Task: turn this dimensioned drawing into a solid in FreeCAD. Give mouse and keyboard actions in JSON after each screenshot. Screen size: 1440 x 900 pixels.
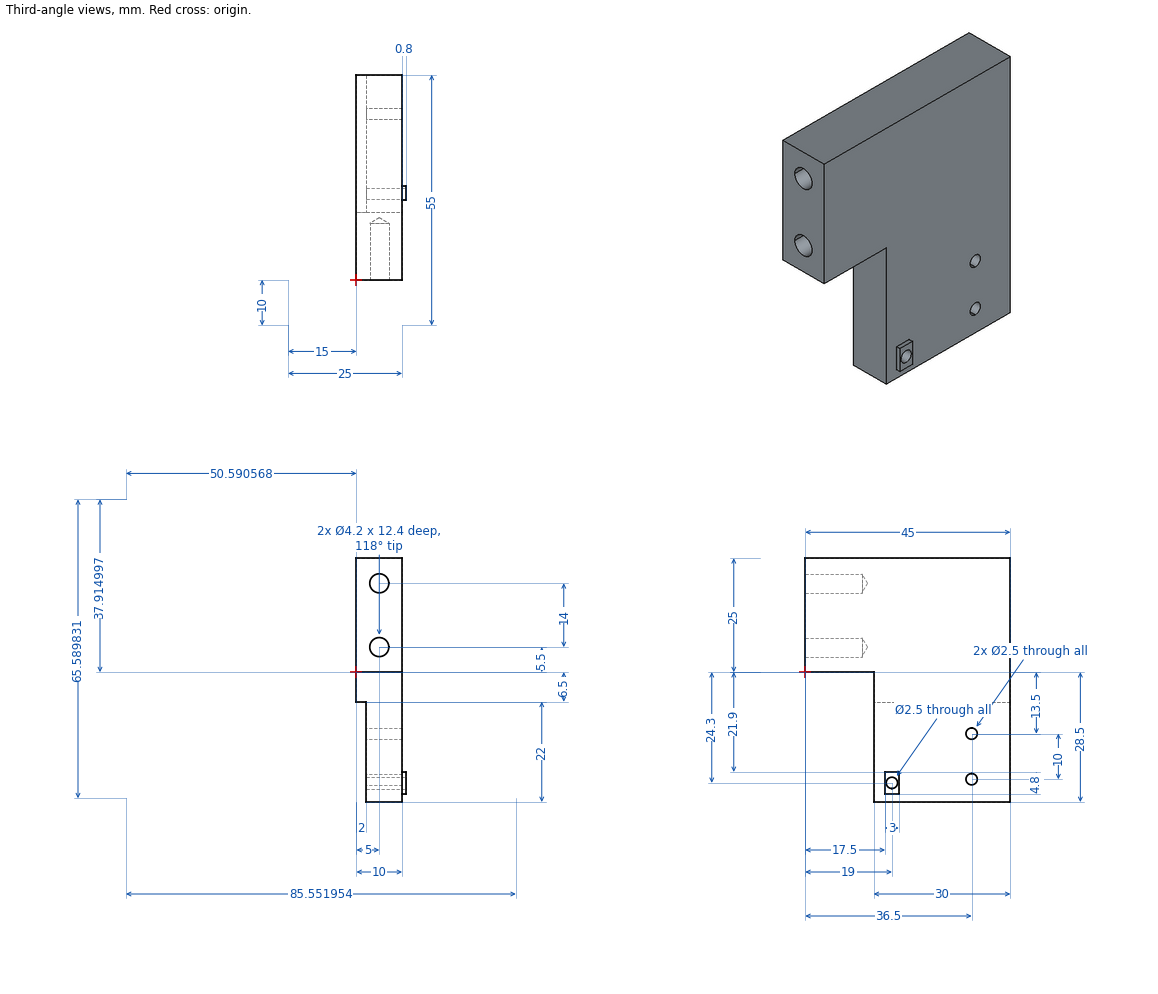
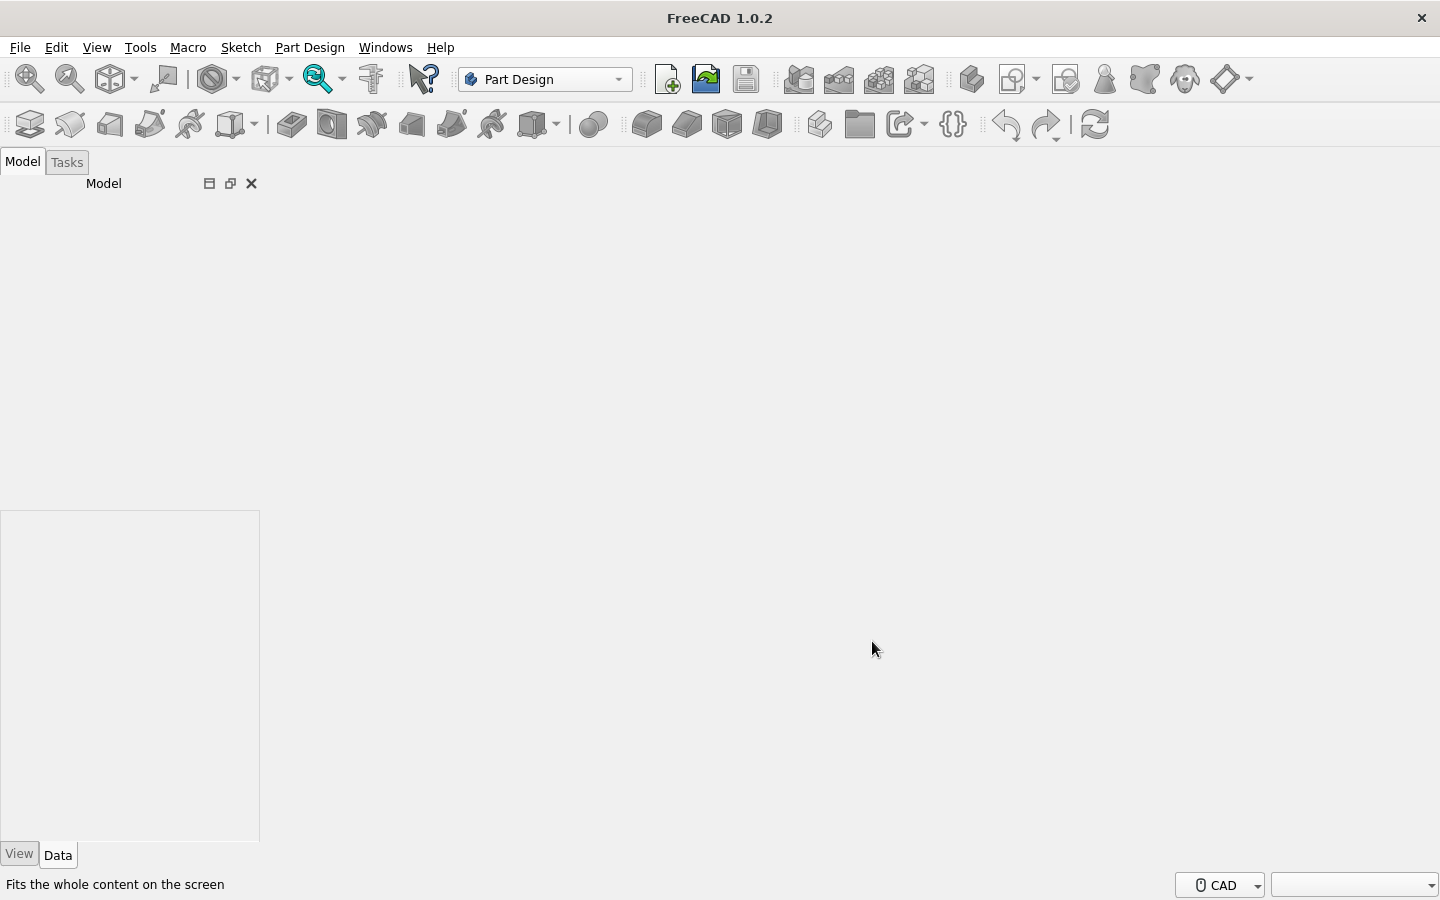
{"action": "left_click", "coordinate": [666, 80]}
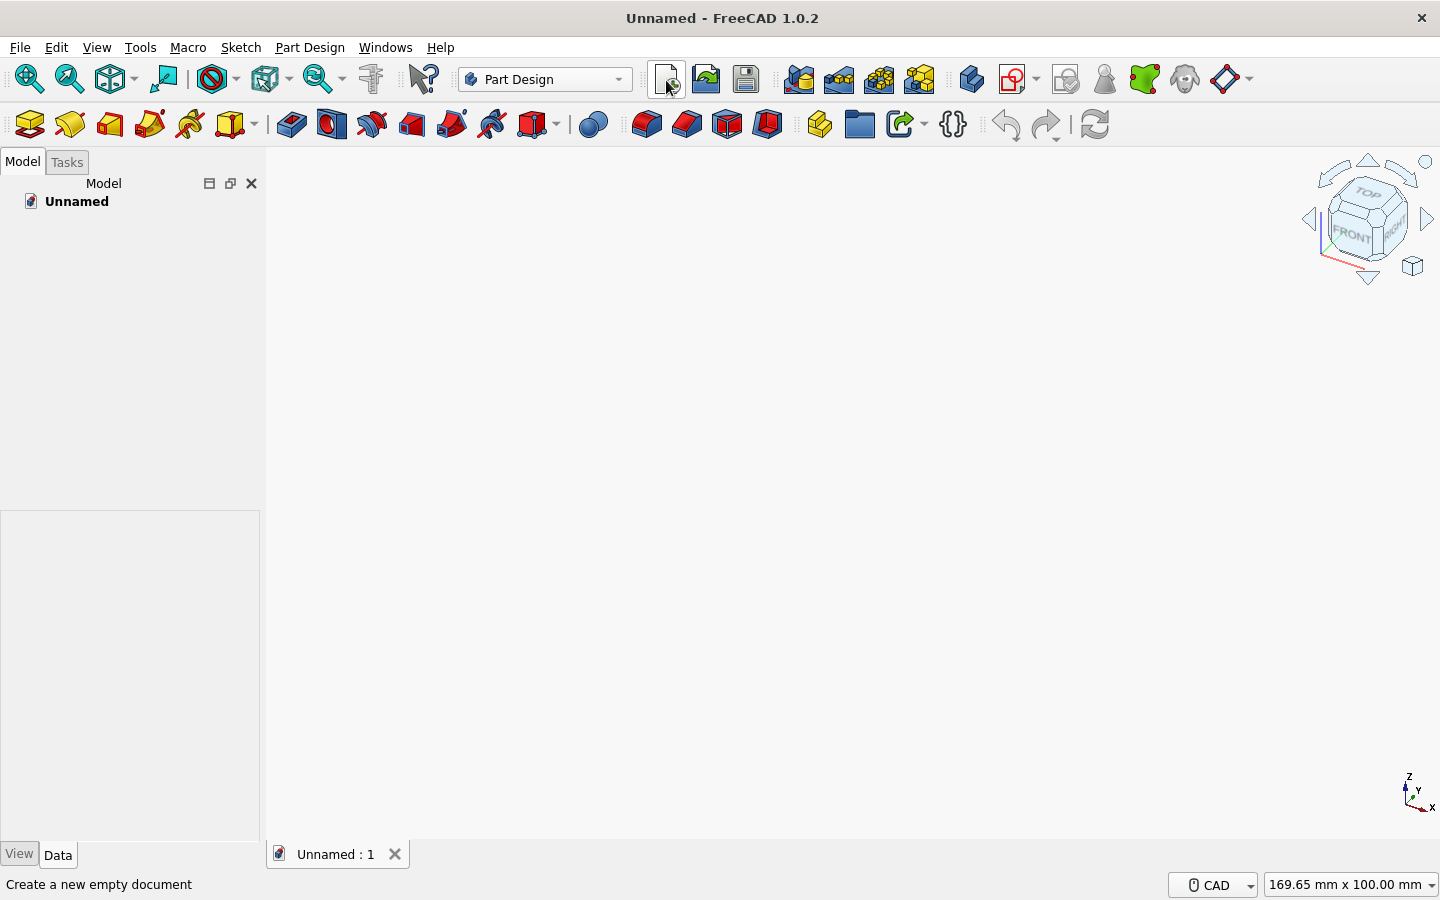
{"action": "left_click", "coordinate": [1012, 80]}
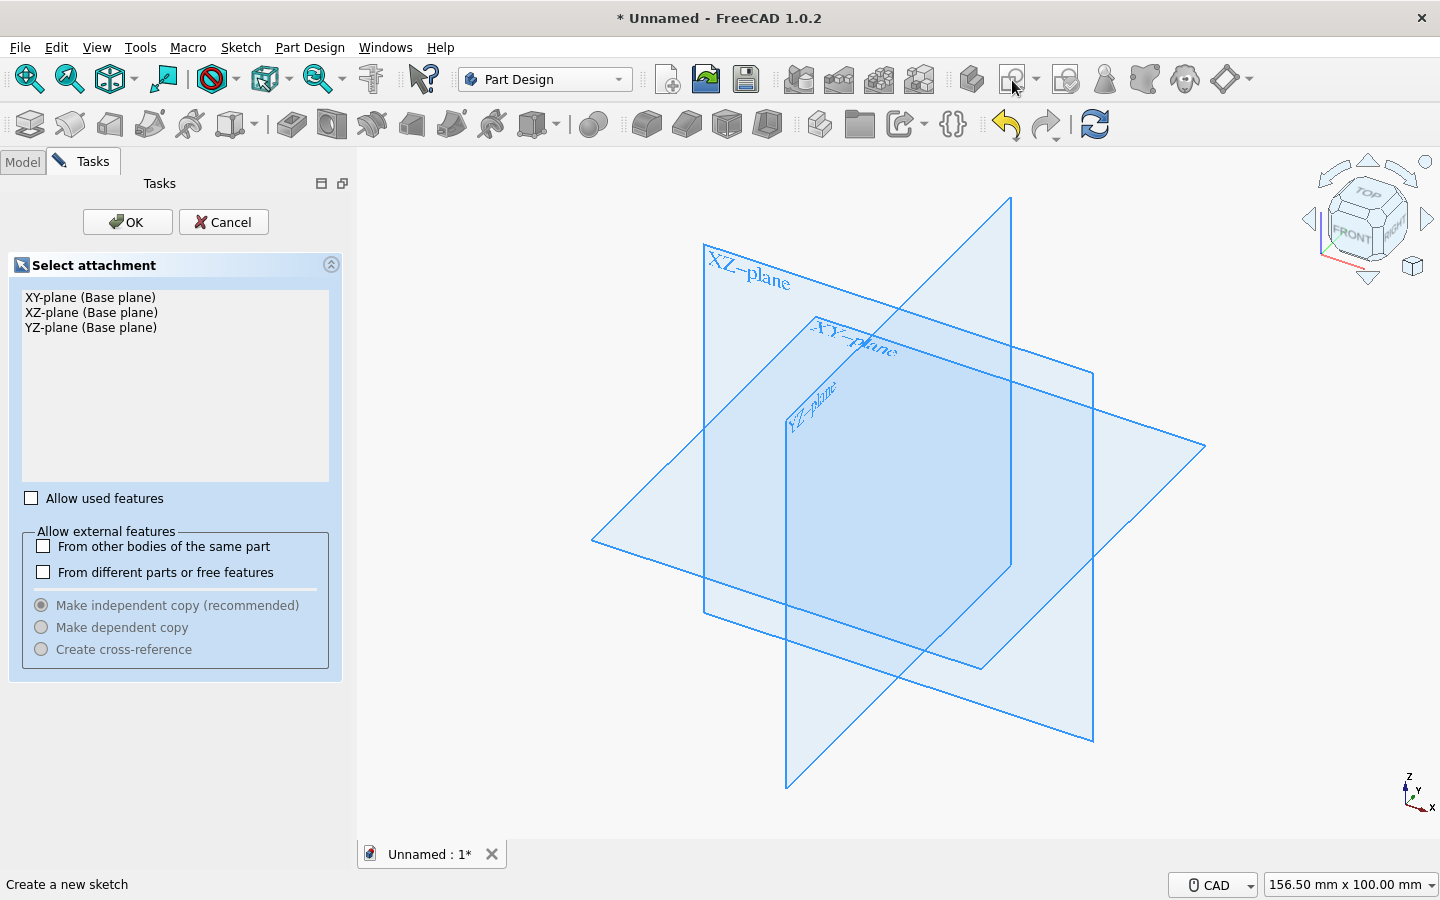
{"action": "left_click", "coordinate": [82, 298]}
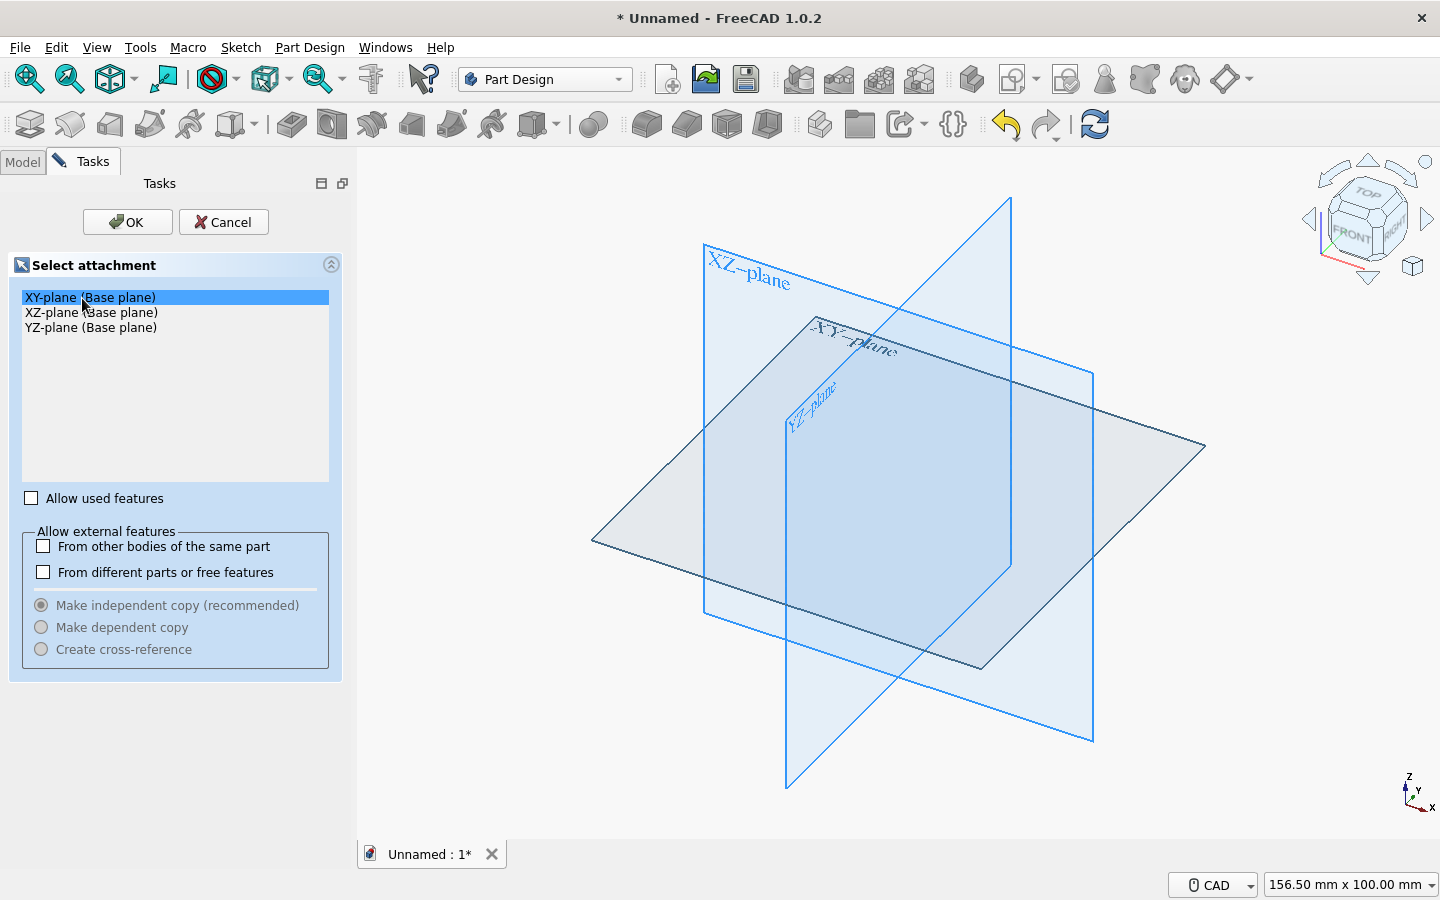
{"action": "left_click", "coordinate": [128, 222]}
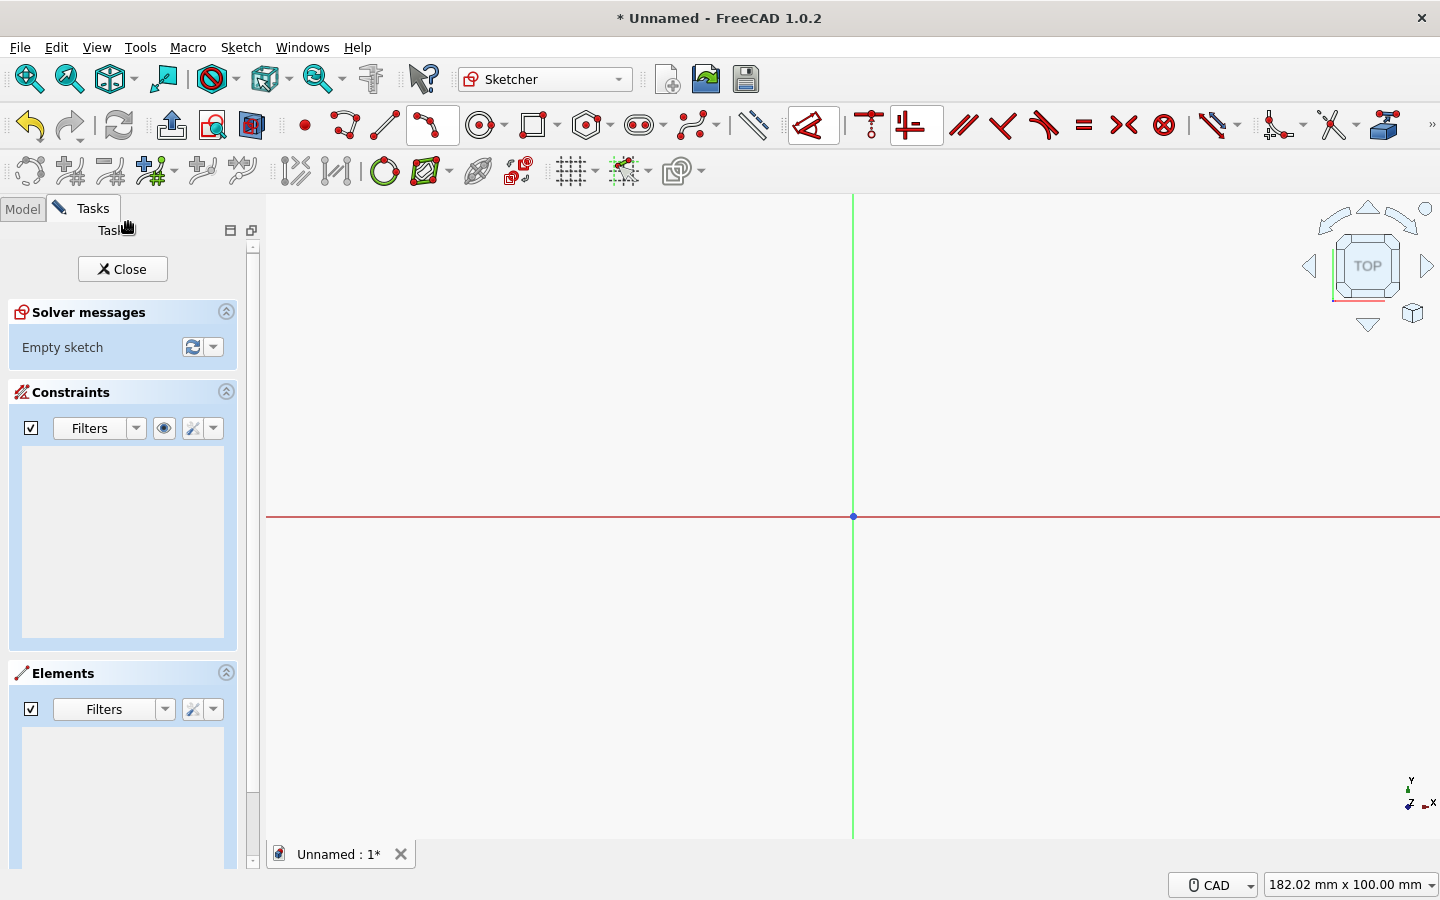
{"action": "scroll", "coordinate": [548, 811], "scroll_direction": "down", "scroll_amount": 1}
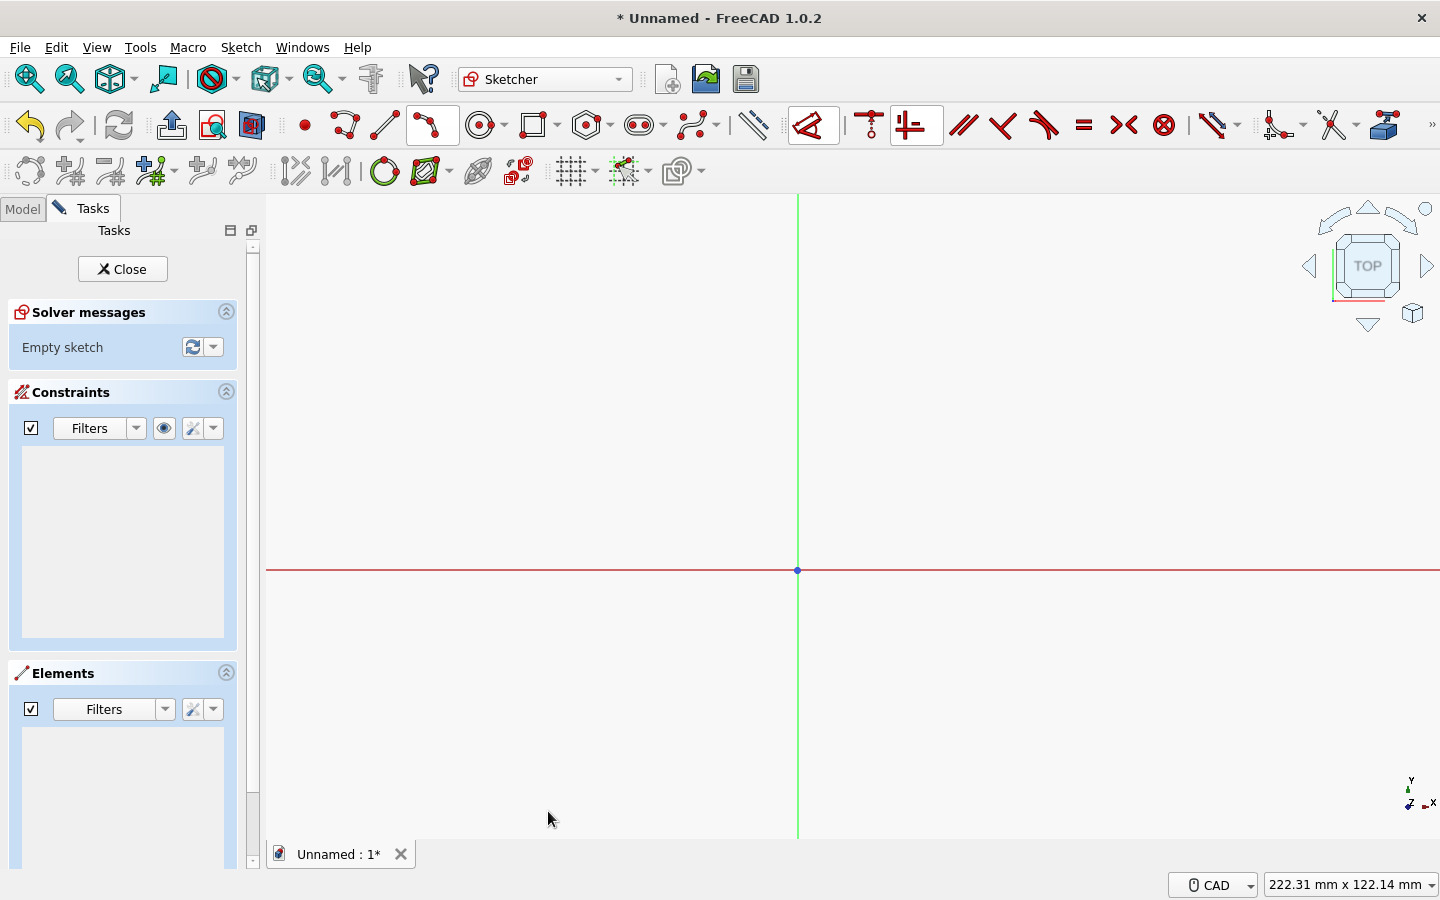
{"action": "scroll", "coordinate": [785, 399], "scroll_direction": "up", "scroll_amount": 2}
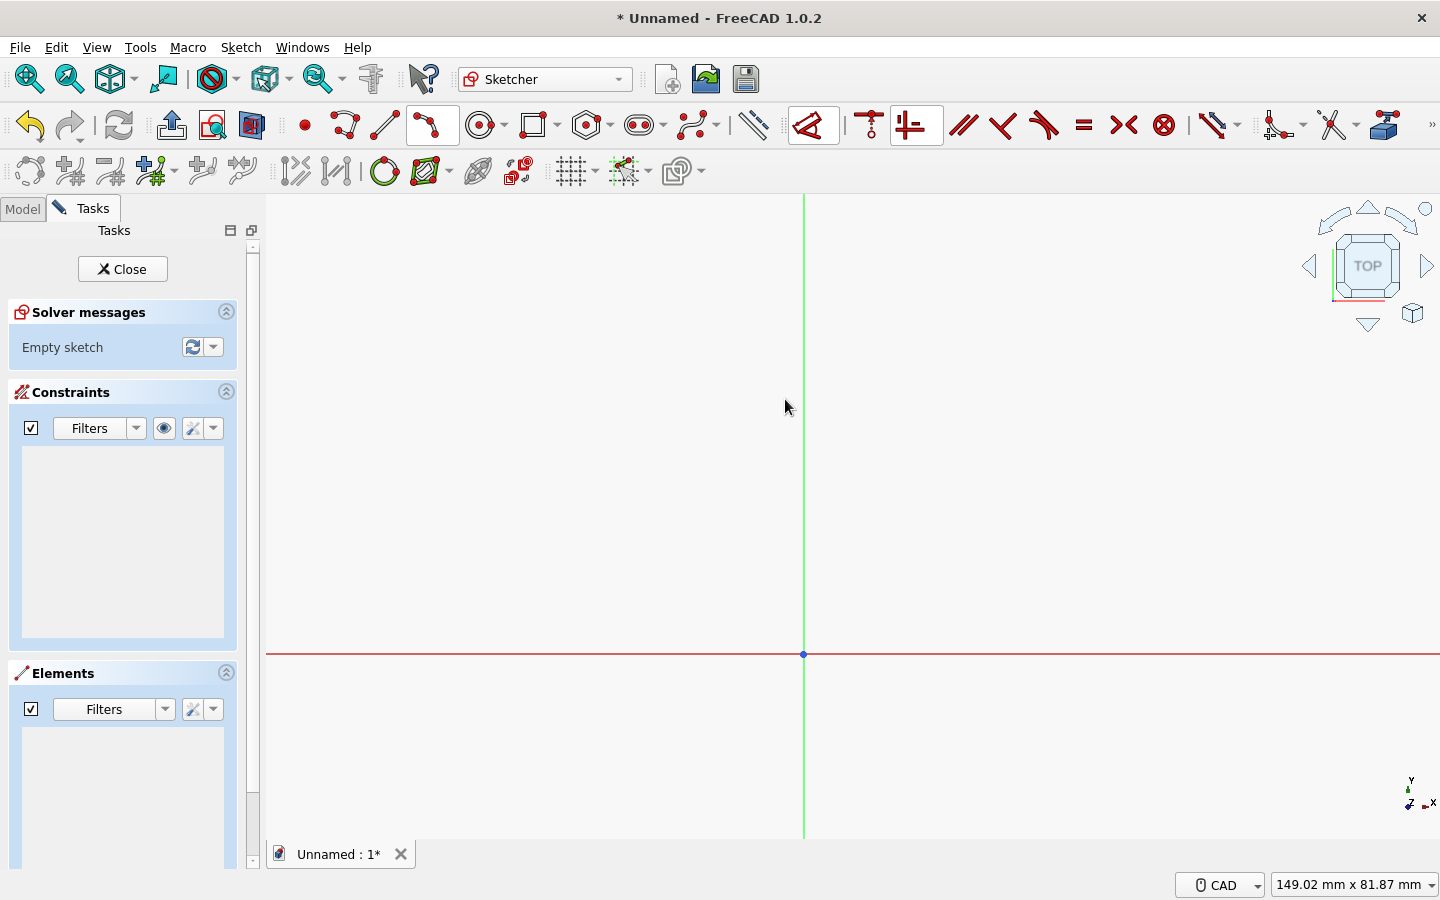
{"action": "left_click", "coordinate": [346, 126]}